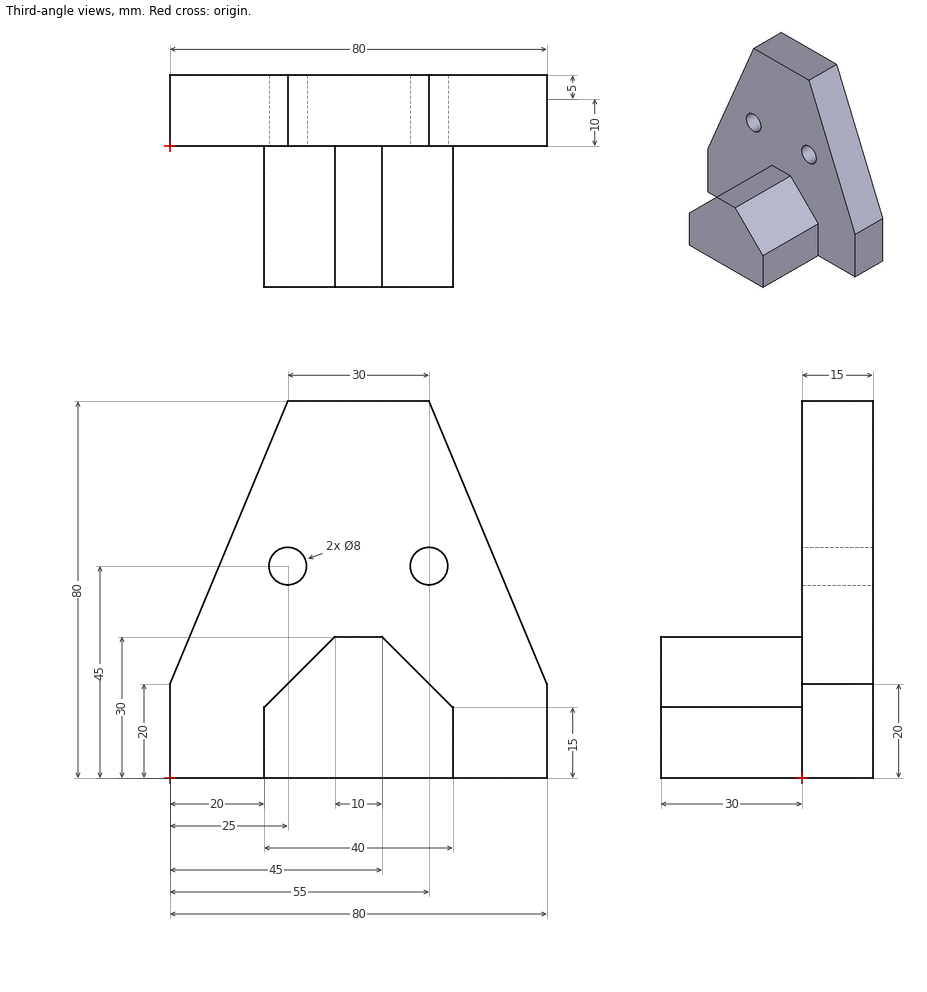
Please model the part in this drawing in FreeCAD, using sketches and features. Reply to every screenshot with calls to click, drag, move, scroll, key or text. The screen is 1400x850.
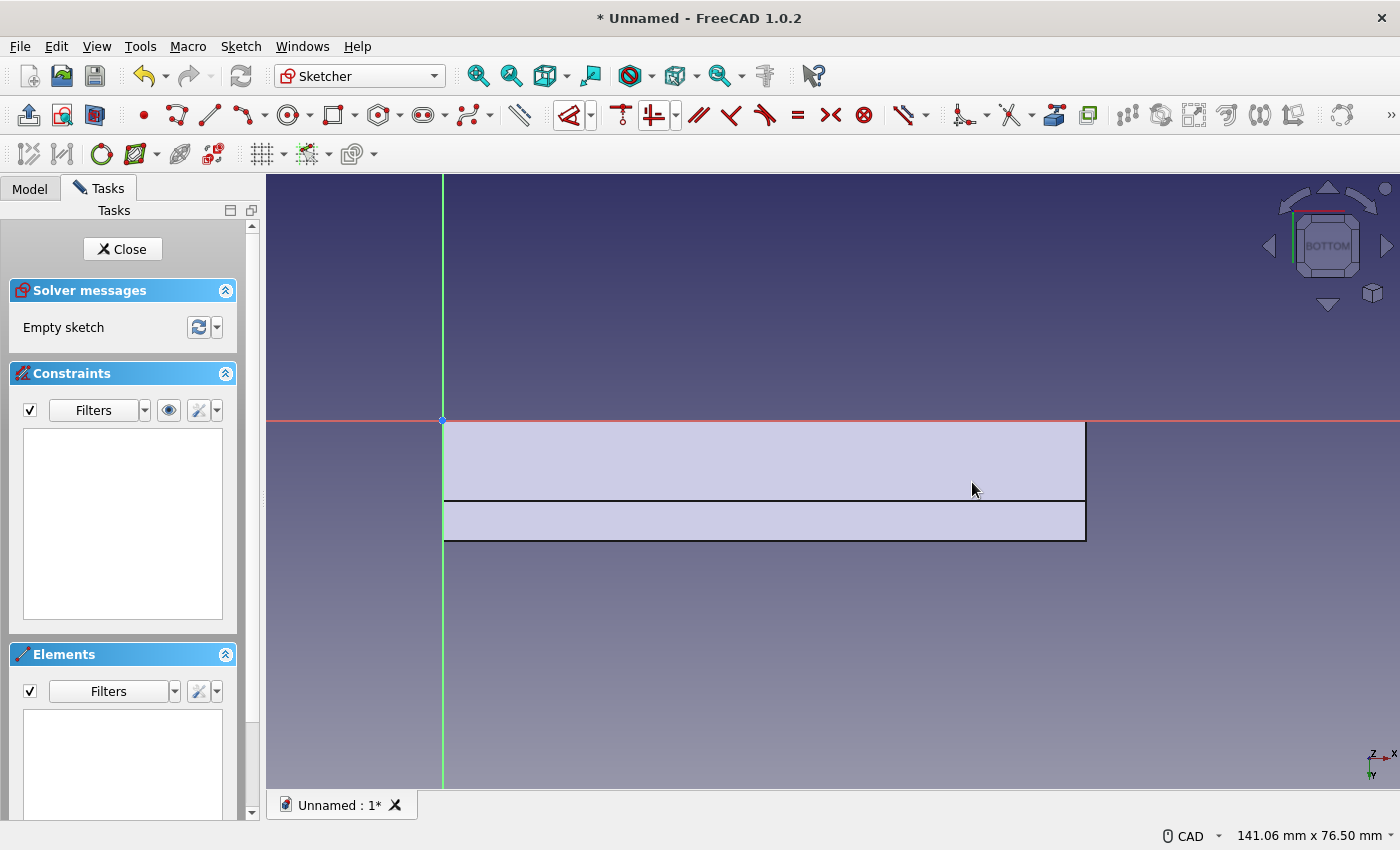
click(332, 116)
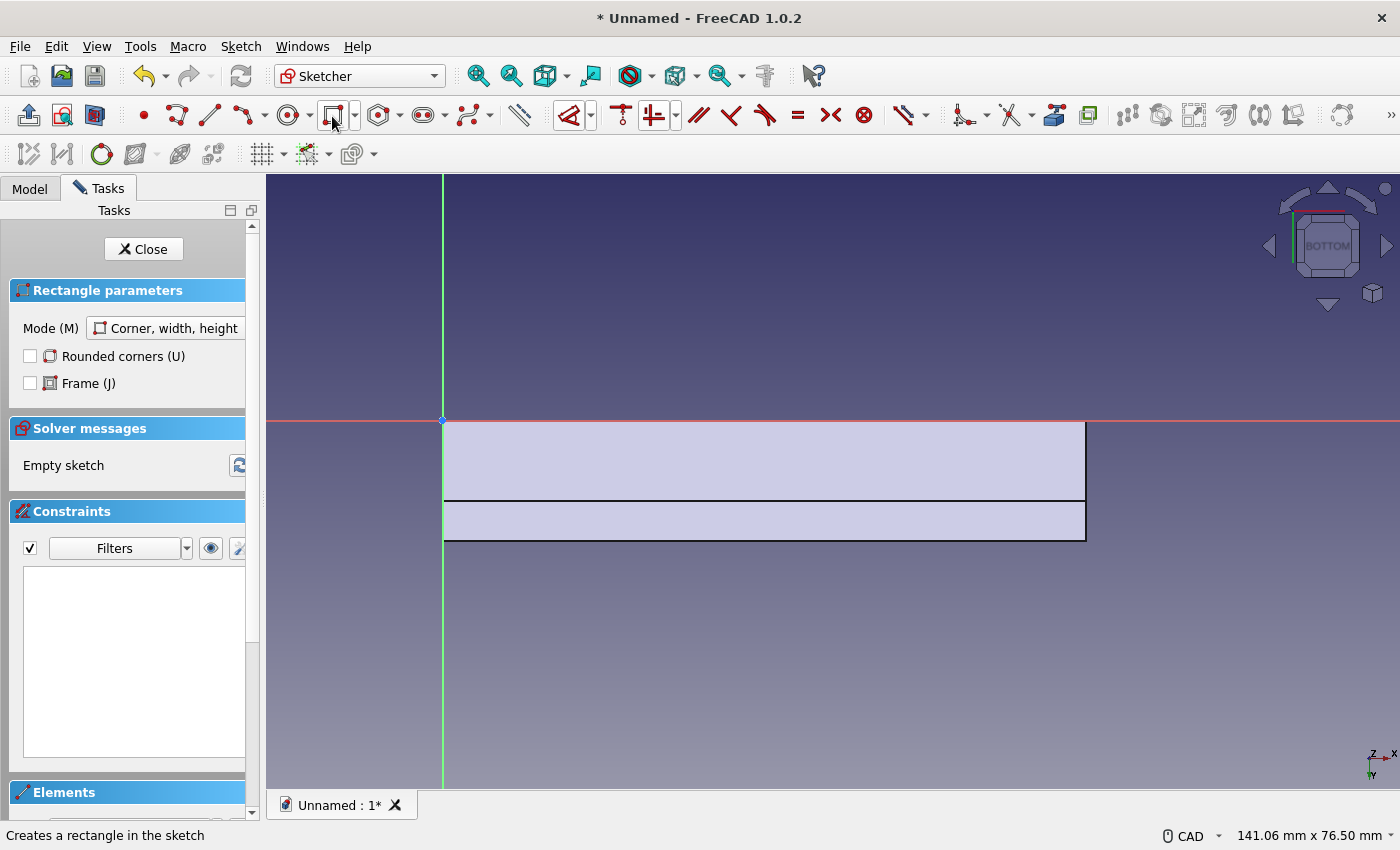
click(443, 501)
move(1086, 541)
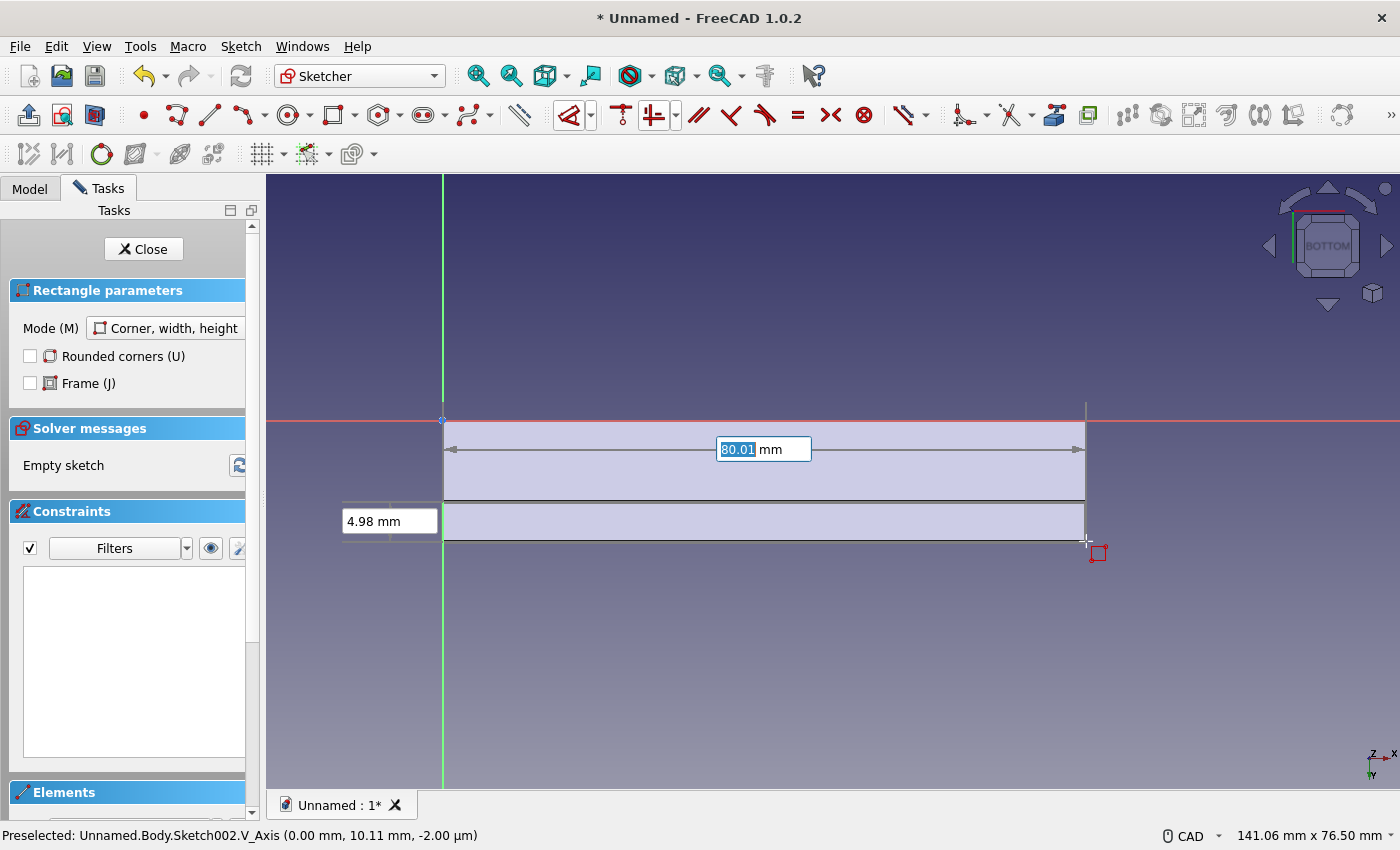
text(80)
key(Tab)
text(5)
key(Return)
key(Escape)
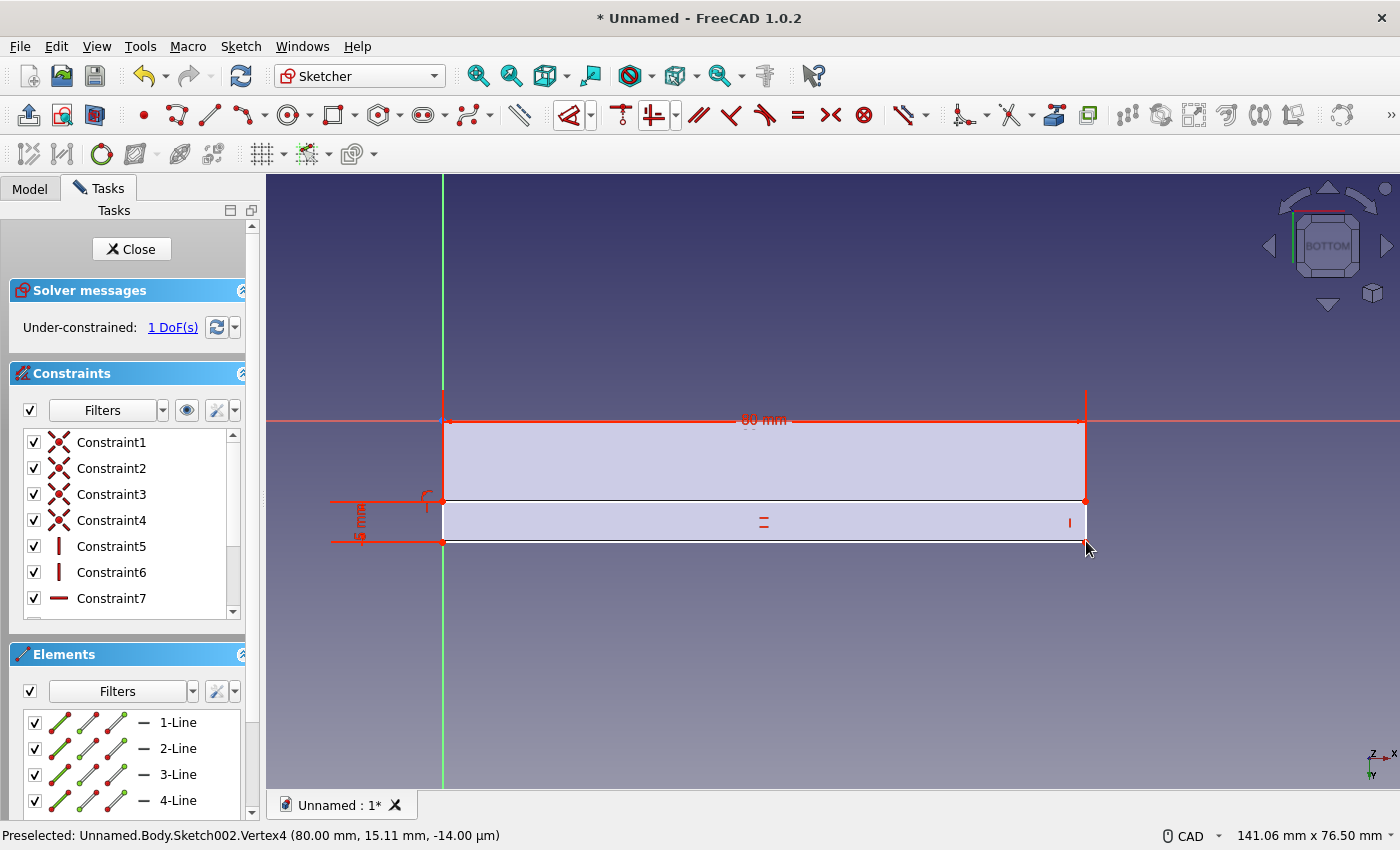
click(443, 502)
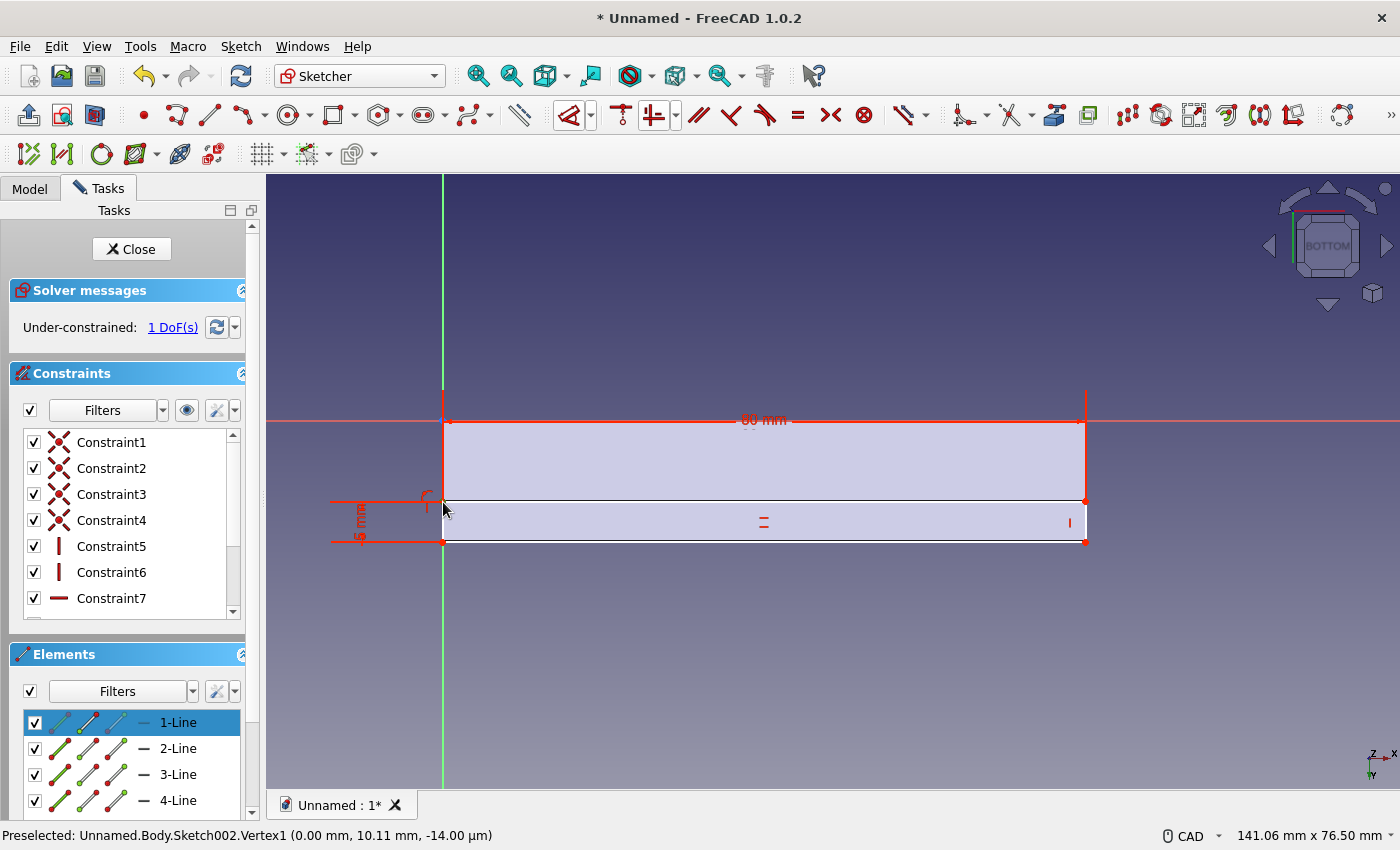
key(i)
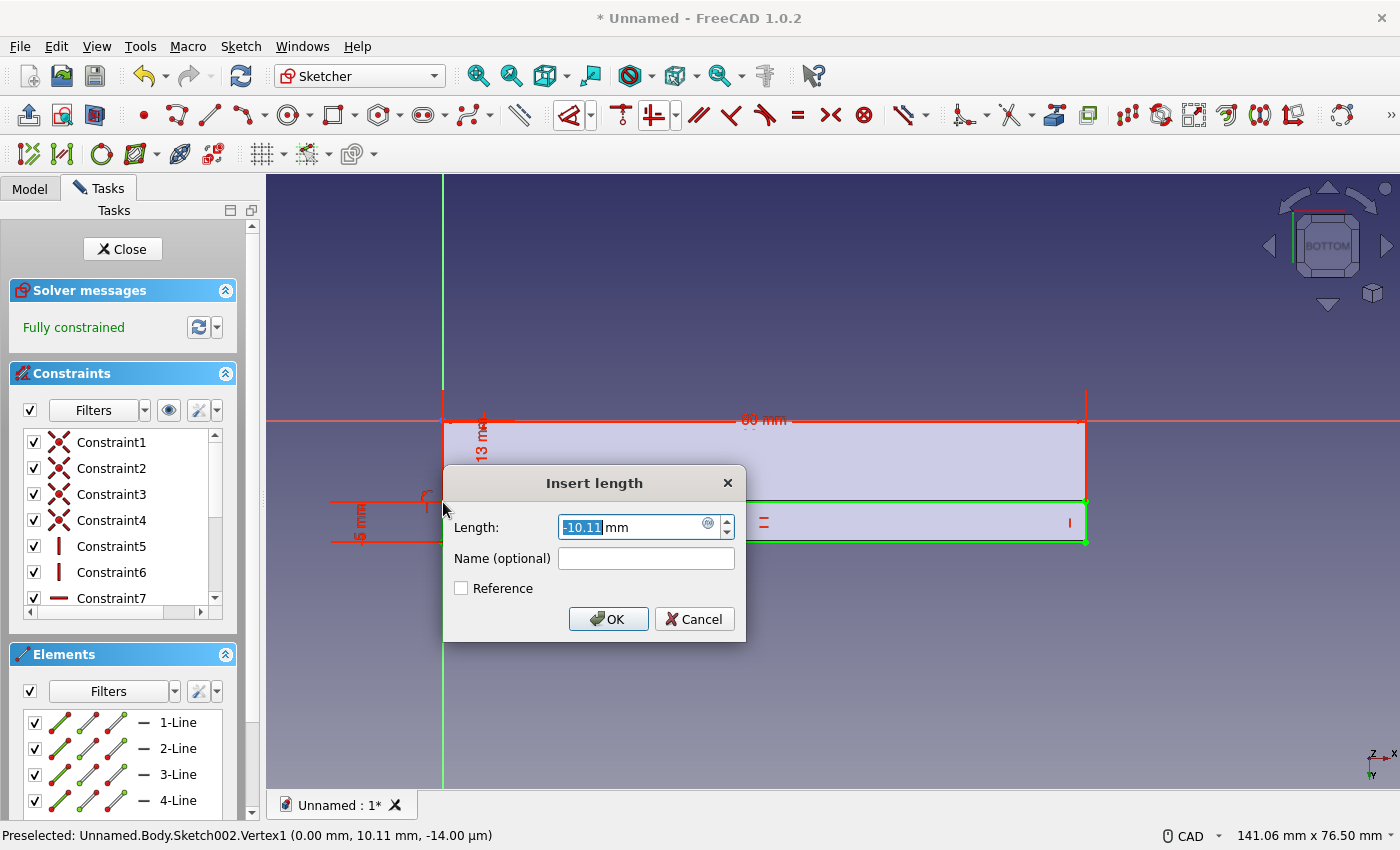
text(-10)
key(Return)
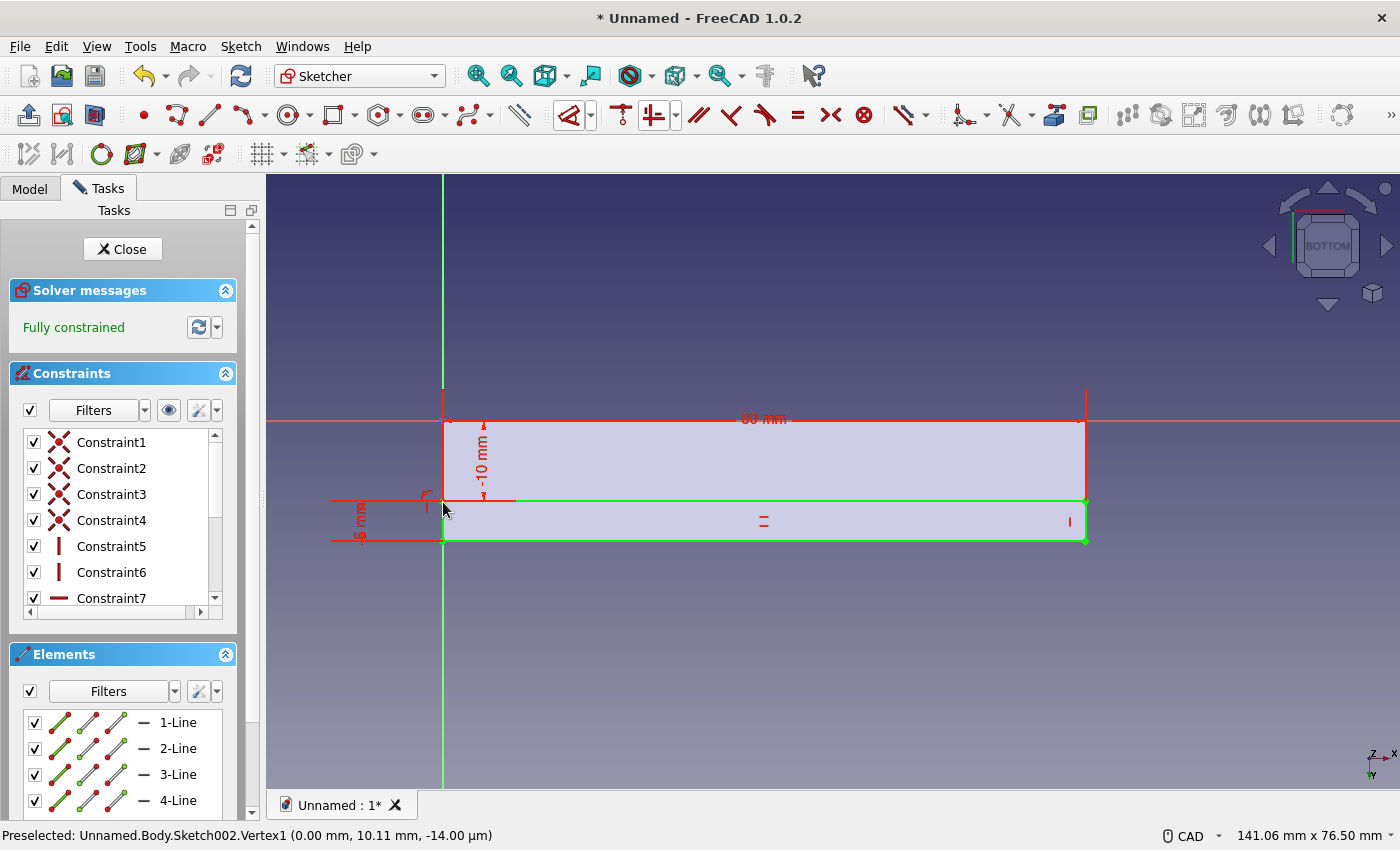
click(123, 249)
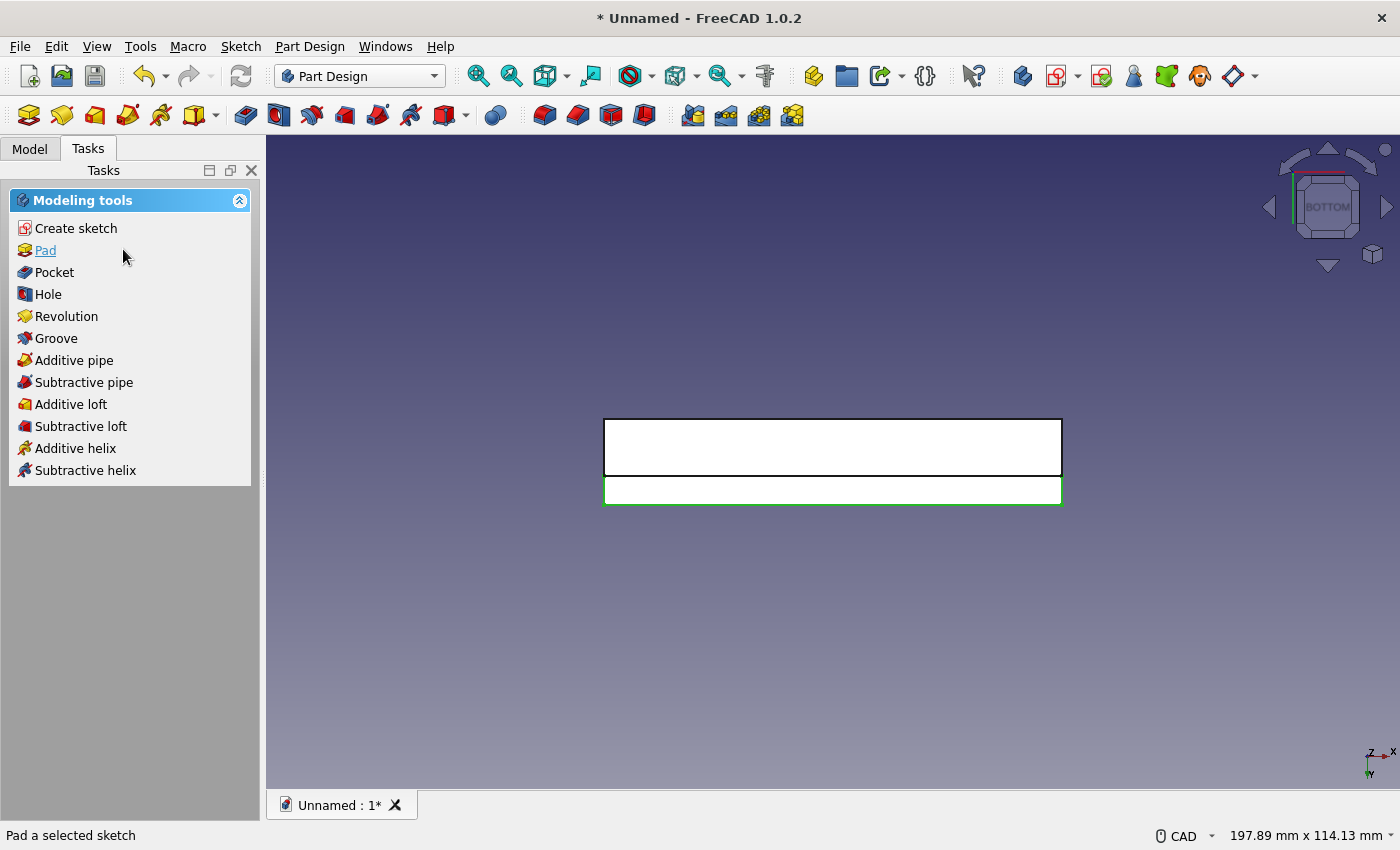
click(29, 116)